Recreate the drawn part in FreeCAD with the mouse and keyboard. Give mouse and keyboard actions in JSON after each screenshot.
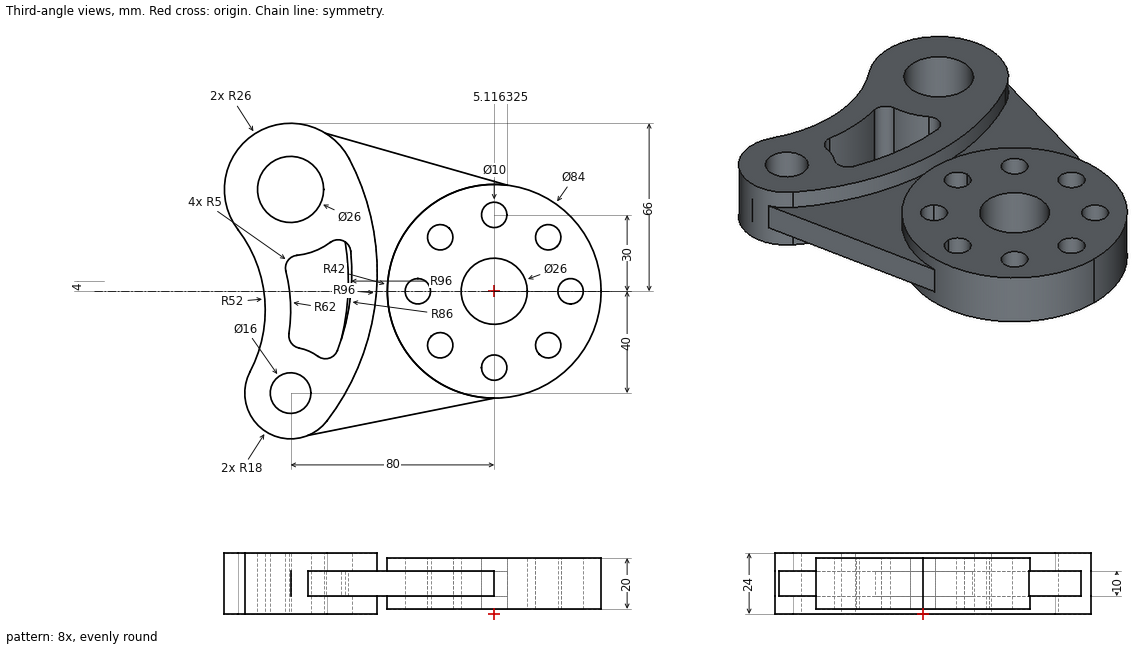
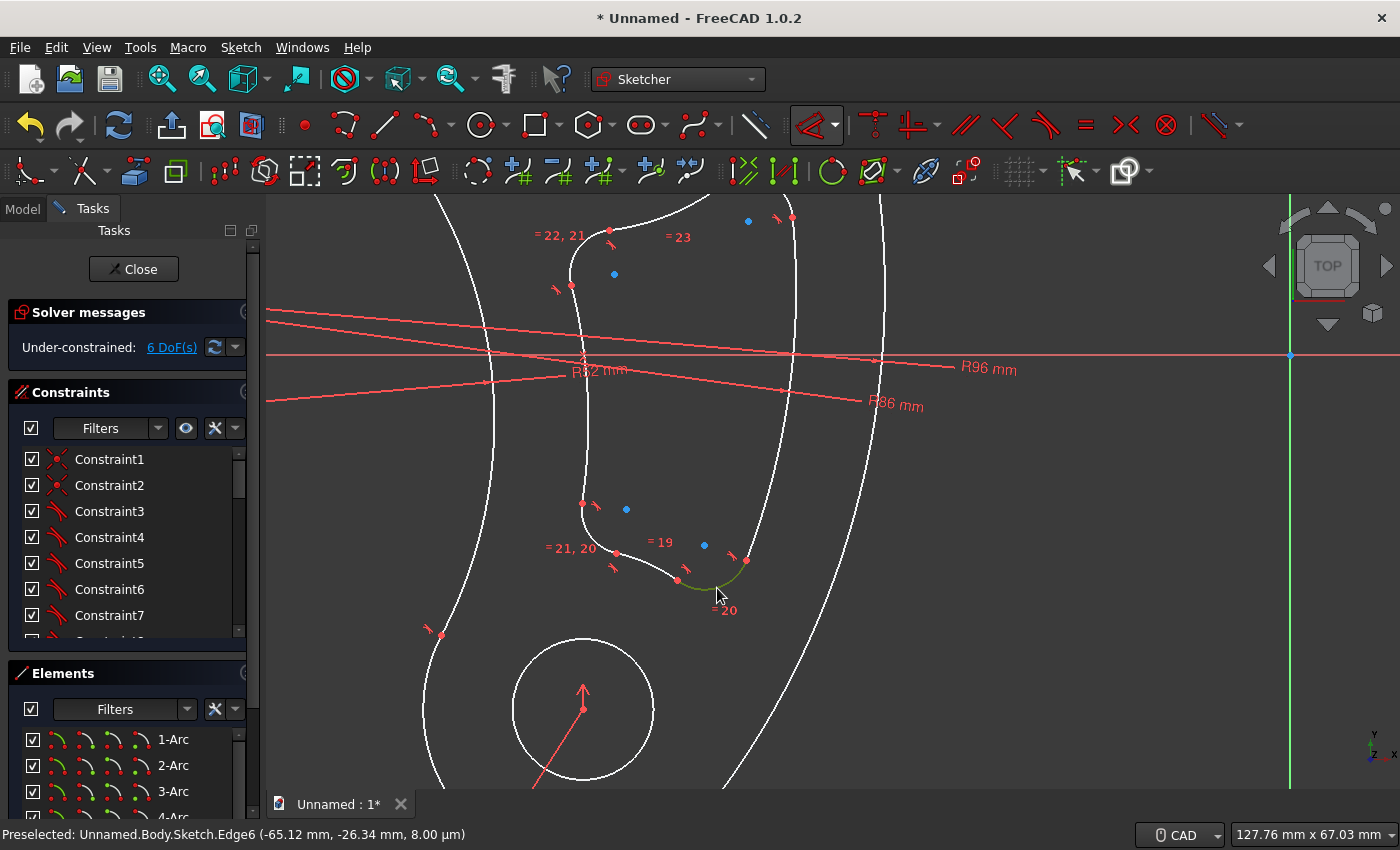
{"action": "key", "text": "k r"}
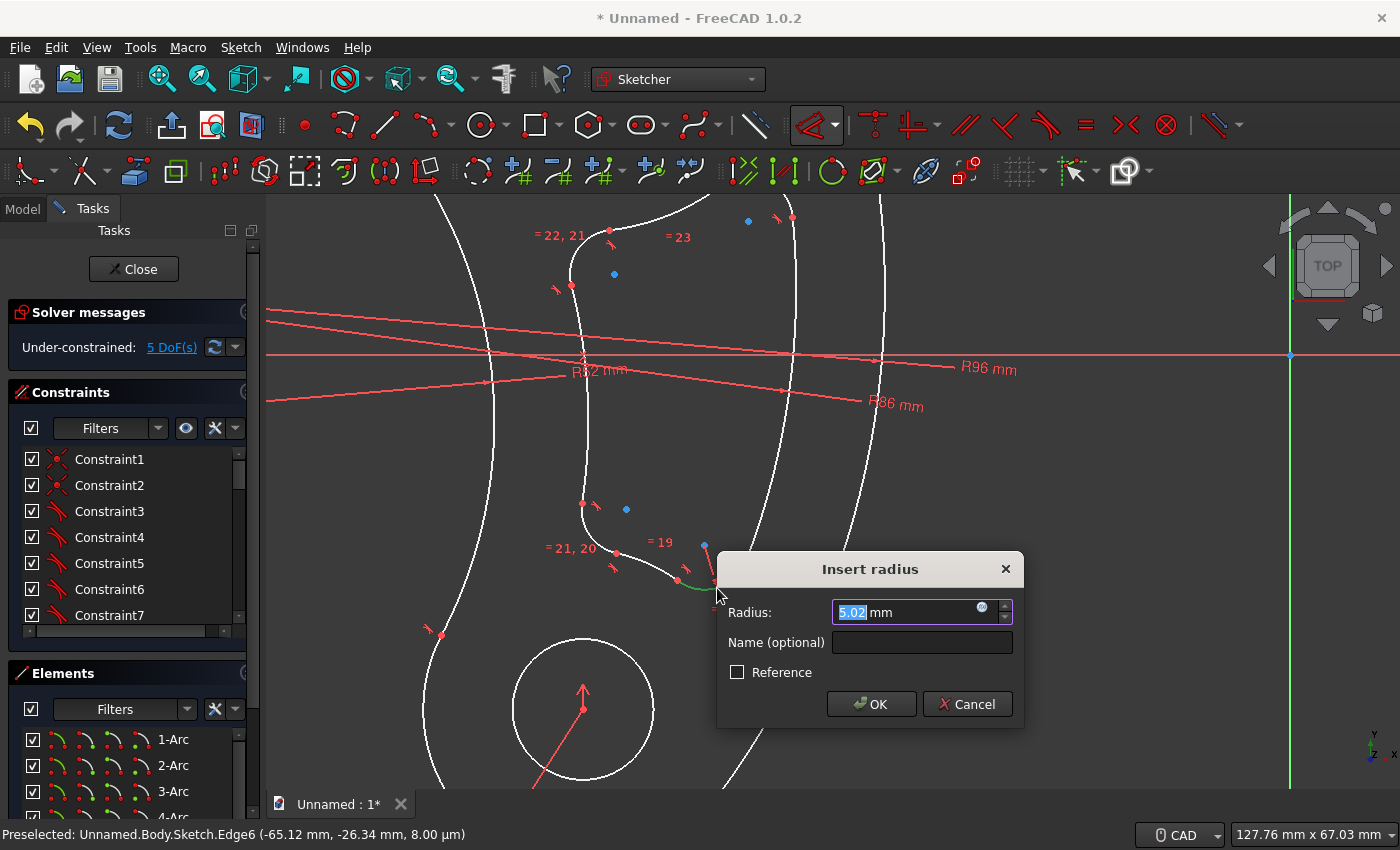
{"action": "type", "text": "5"}
{"action": "key", "text": "Return"}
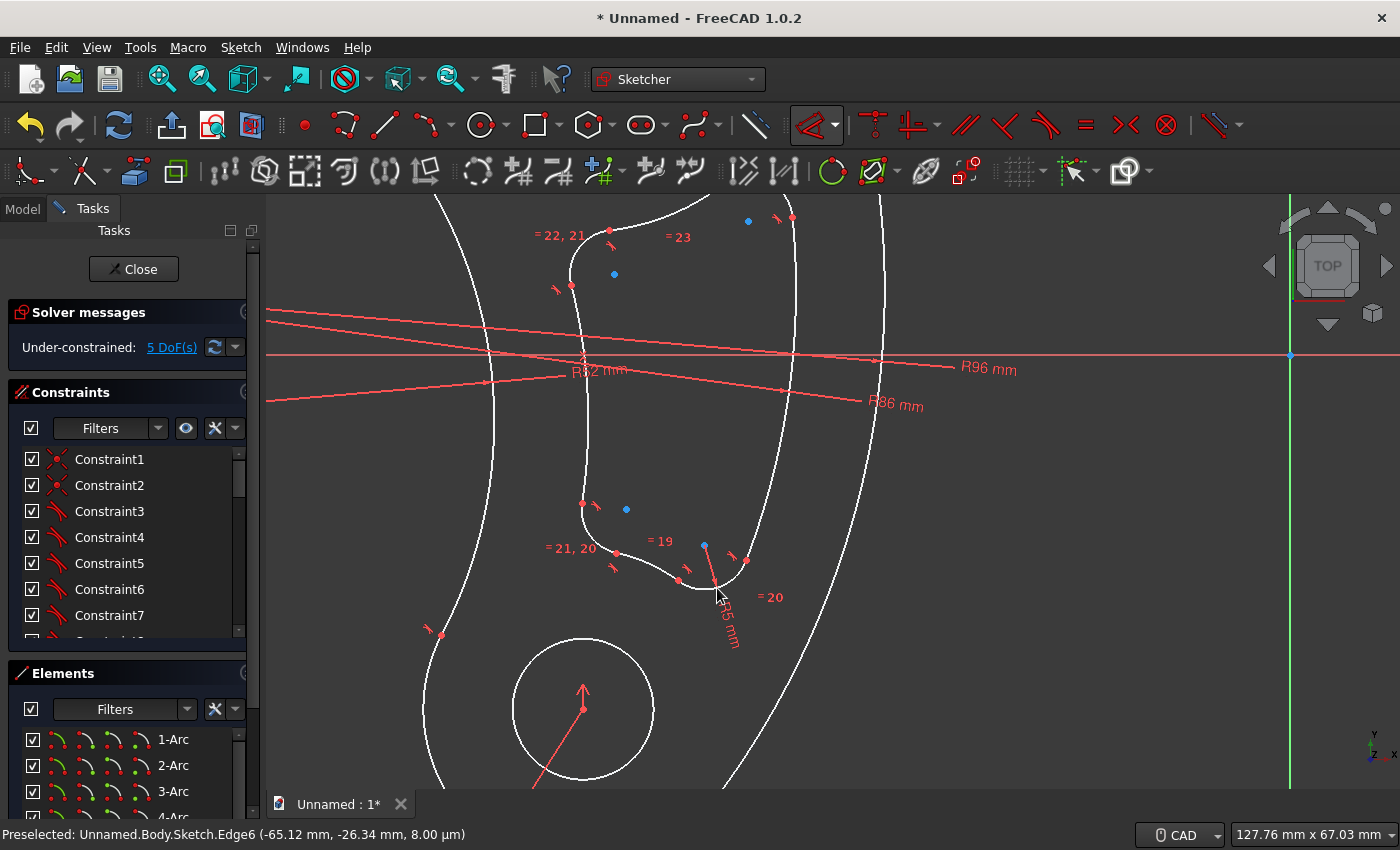
{"action": "left_click", "coordinate": [588, 438]}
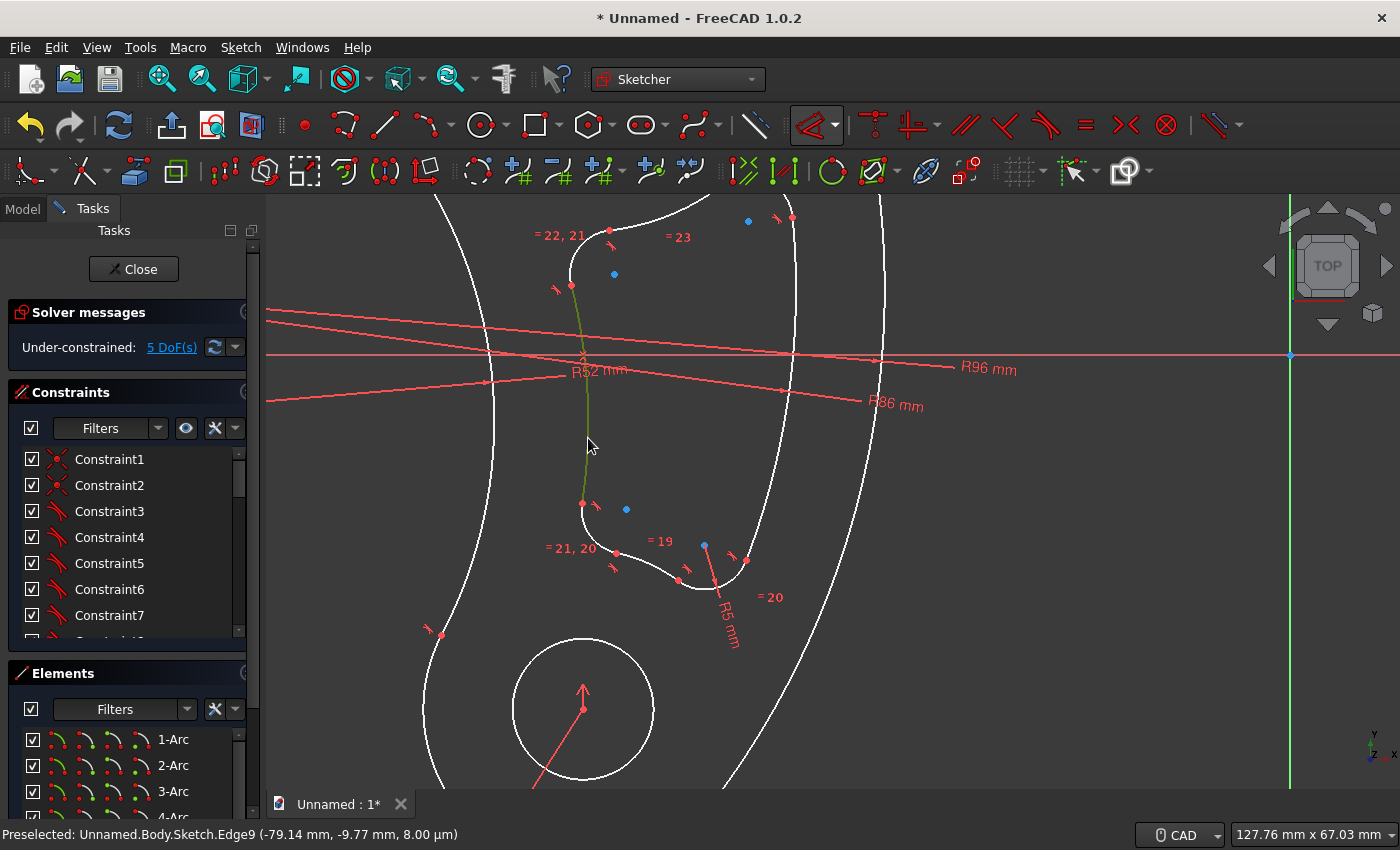
{"action": "key", "text": "k r"}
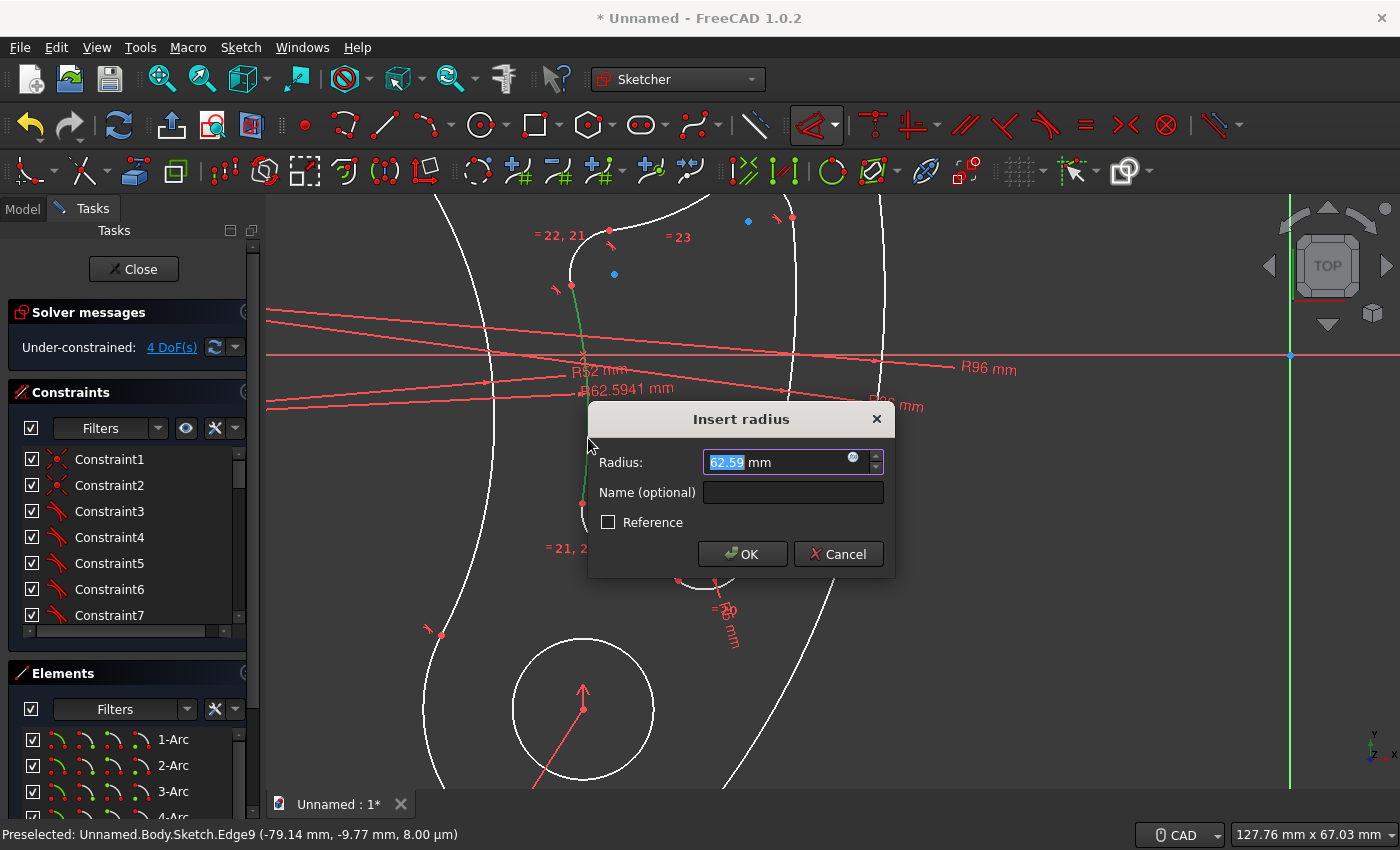
{"action": "type", "text": "62"}
{"action": "key", "text": "Return"}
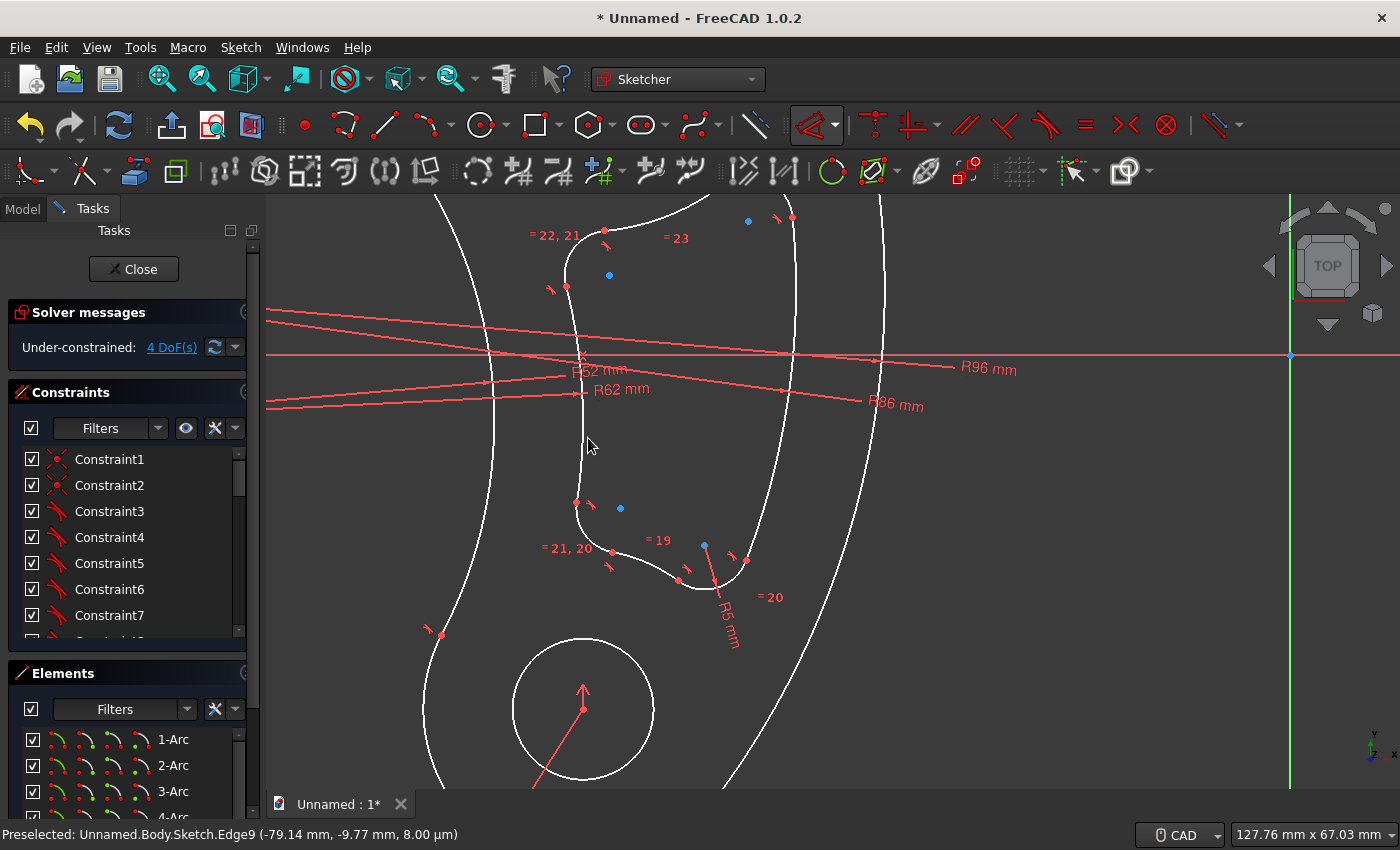
{"action": "left_click", "coordinate": [633, 659]}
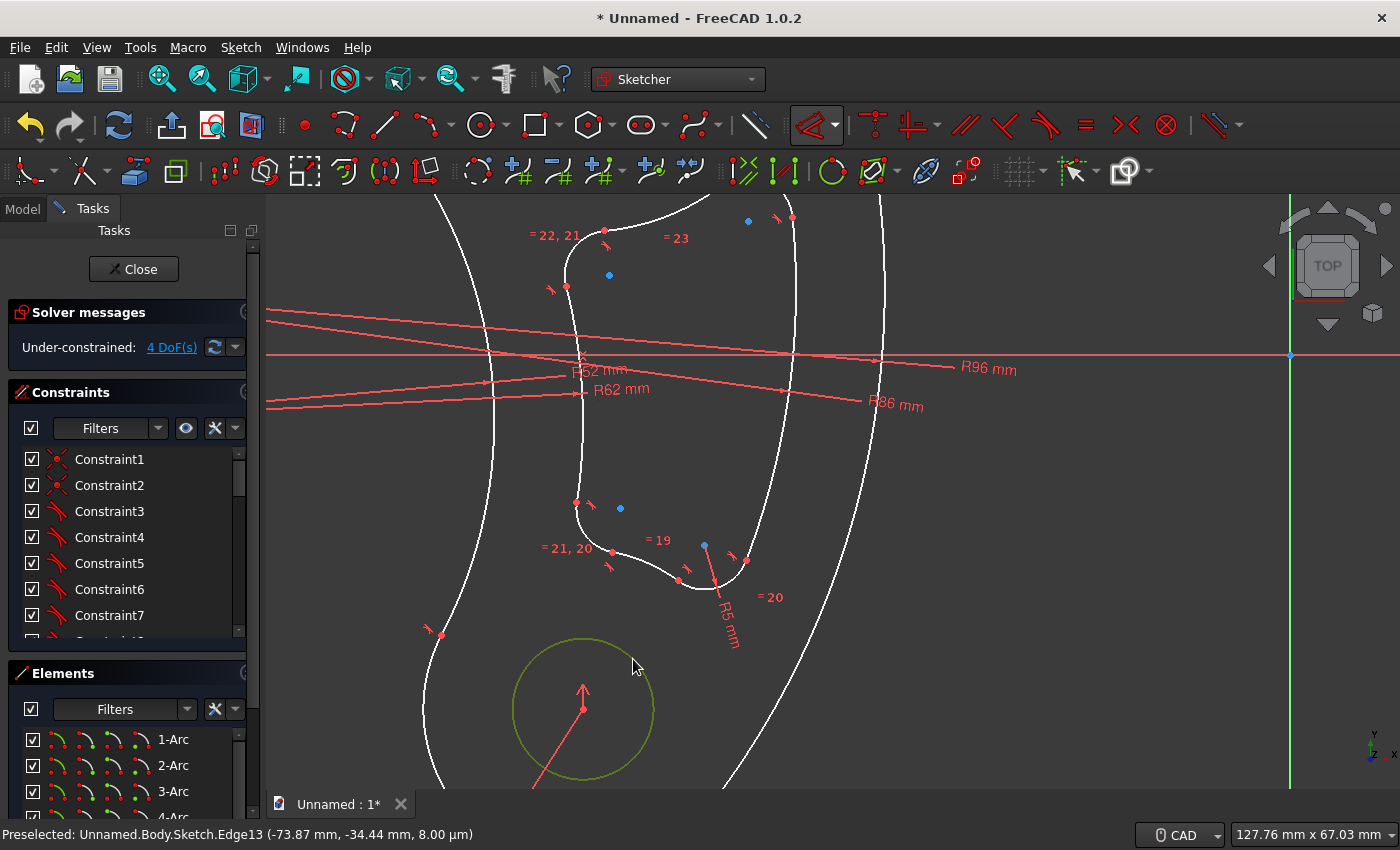
{"action": "key", "text": "k o"}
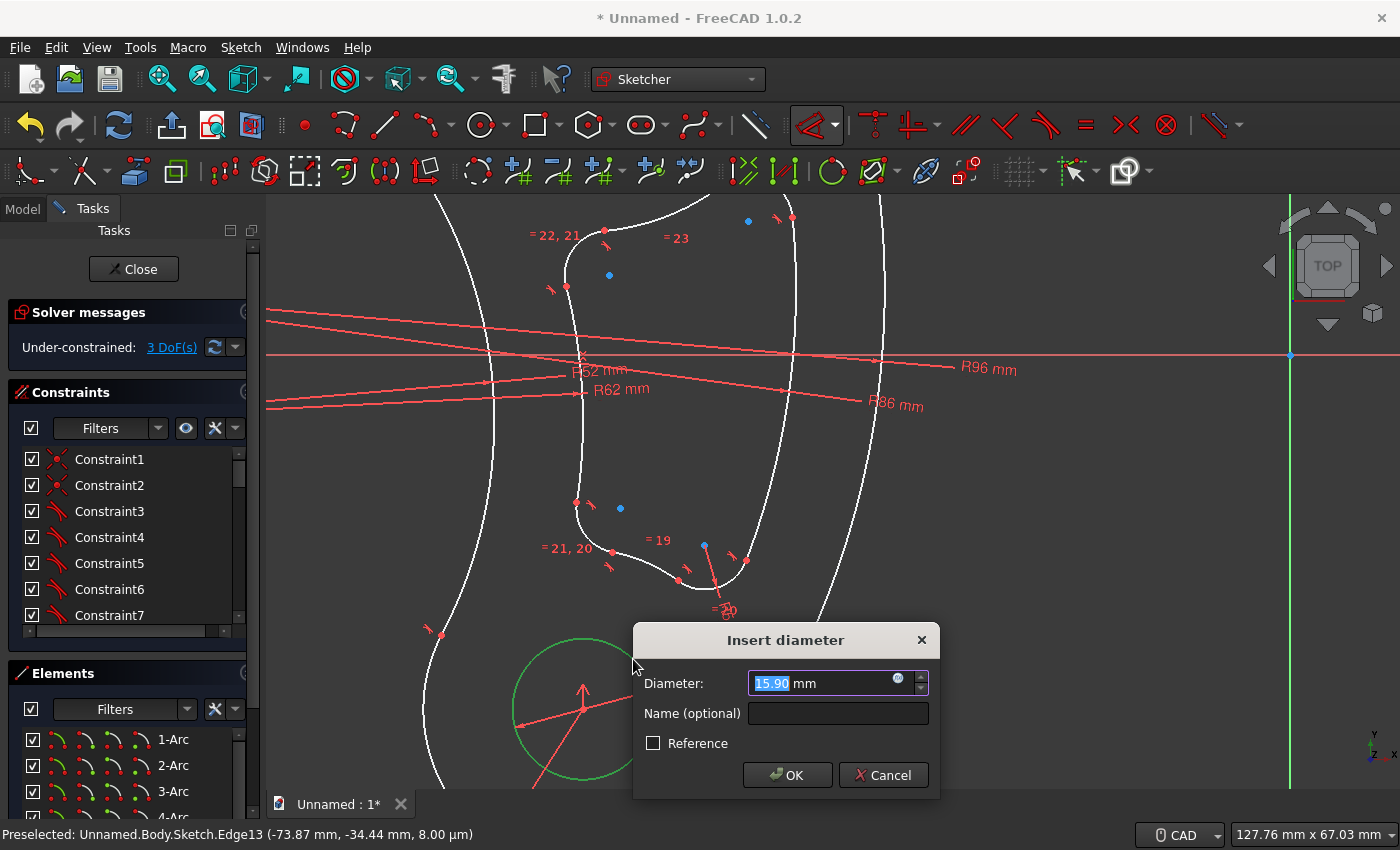
{"action": "type", "text": "16"}
{"action": "key", "text": "Return"}